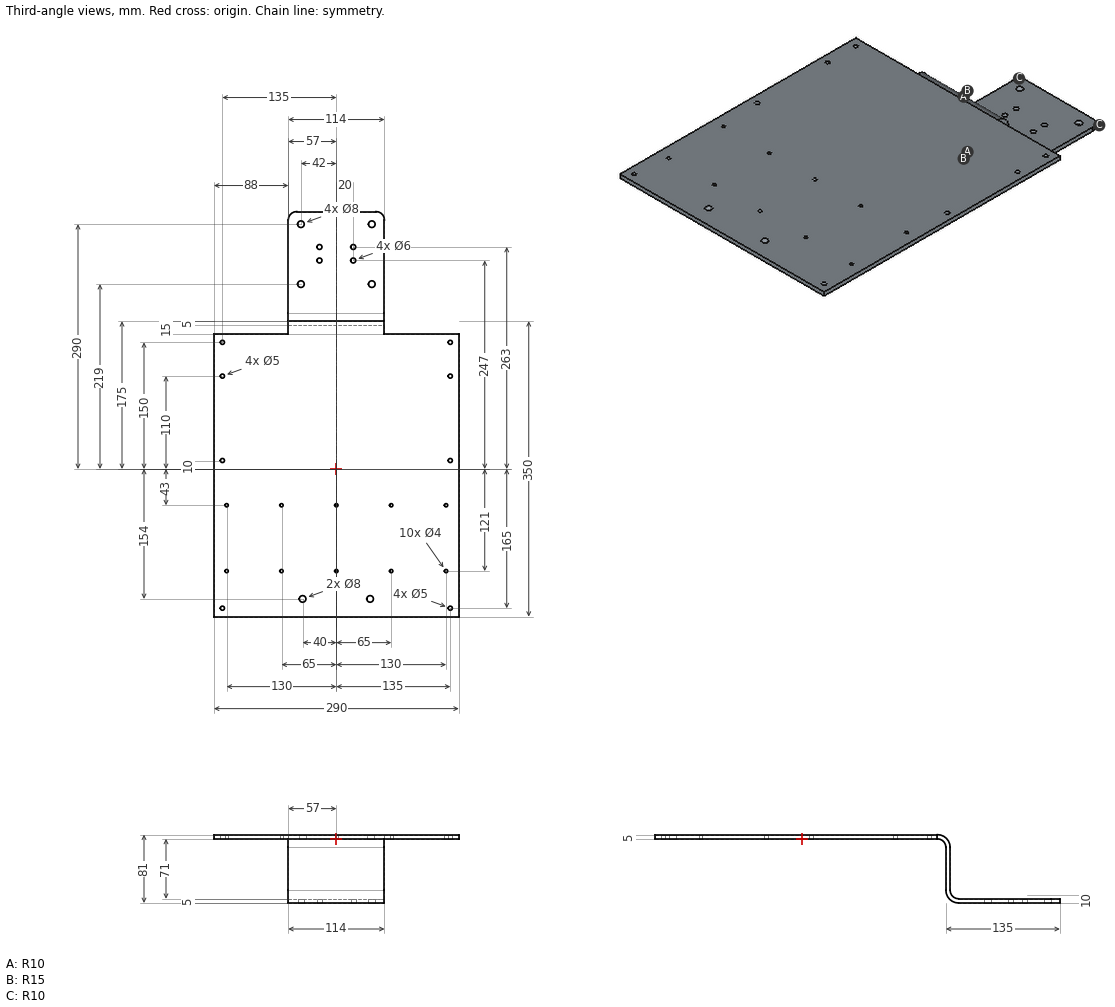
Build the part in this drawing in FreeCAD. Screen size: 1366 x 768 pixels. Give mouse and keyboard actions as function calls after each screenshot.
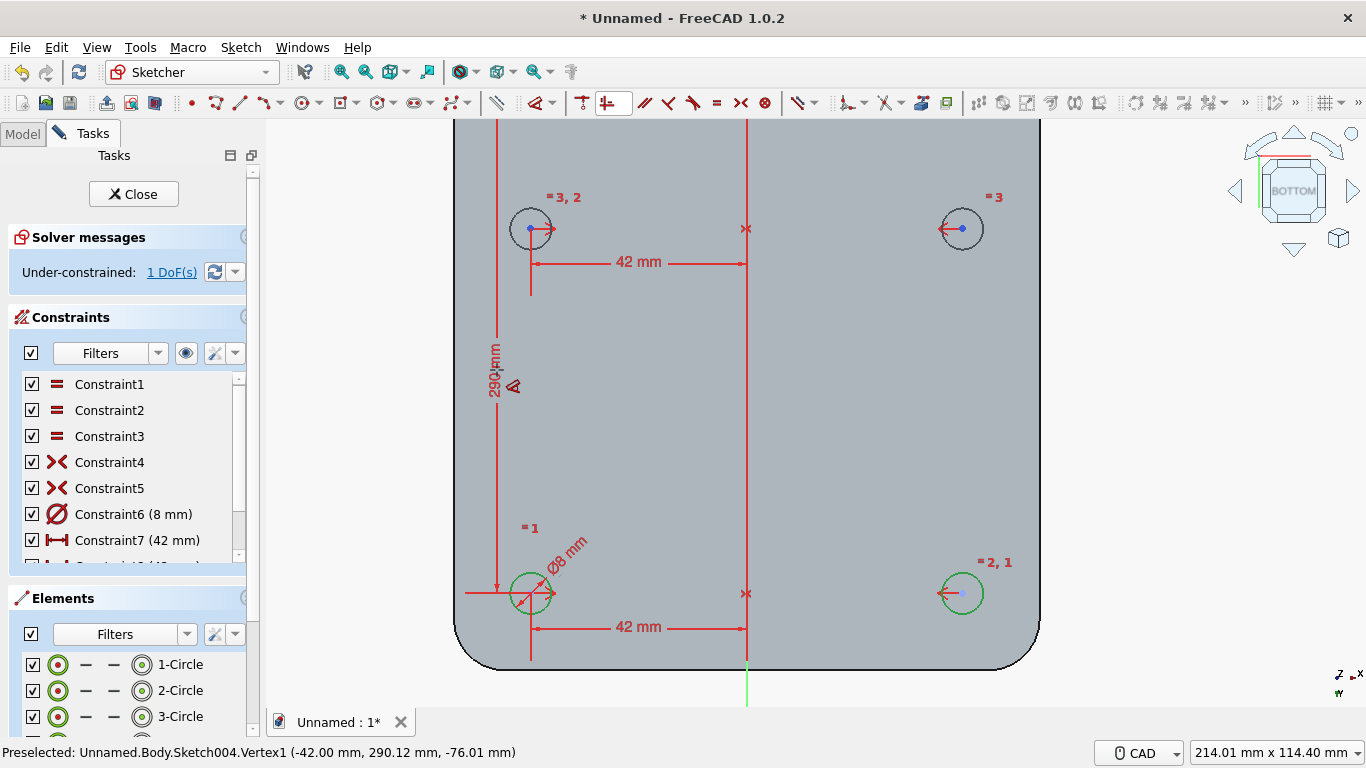
click(531, 229)
click(497, 188)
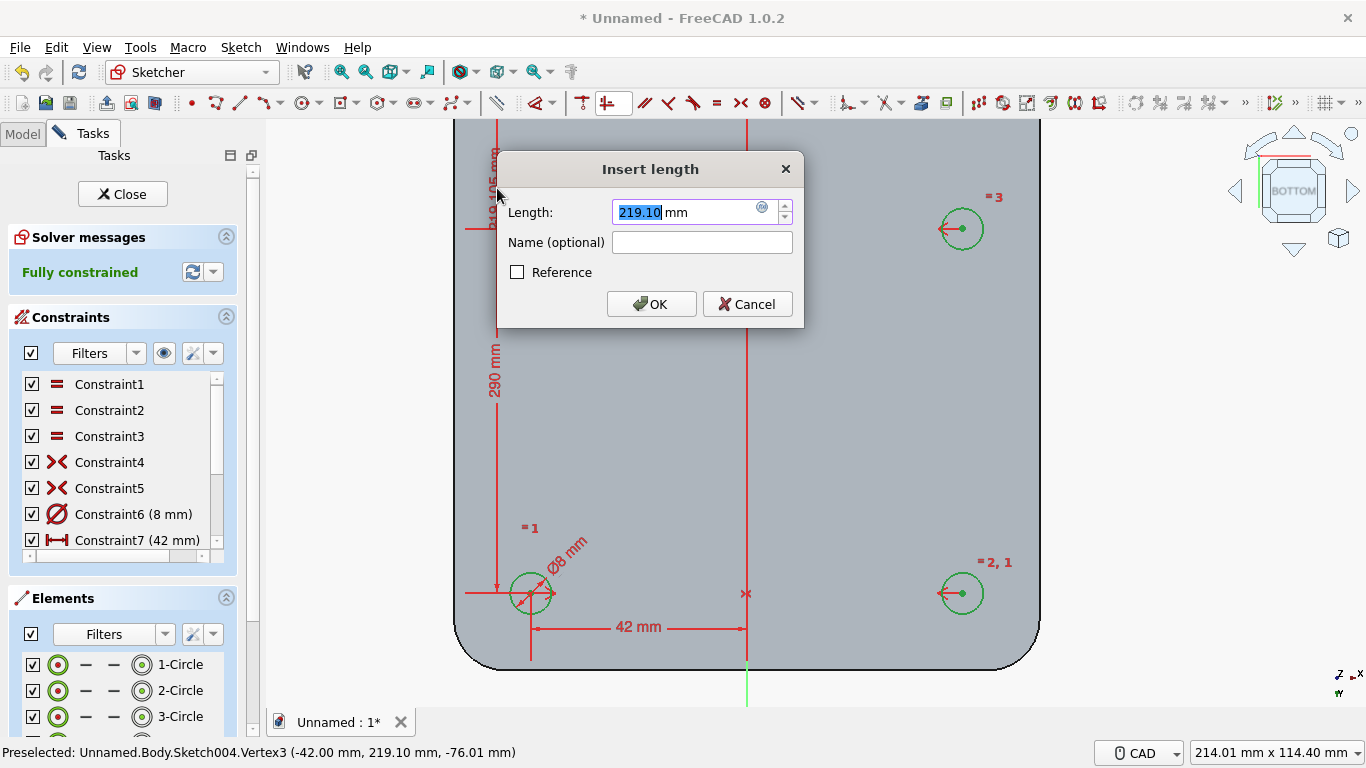
text(219)
key(Return)
key(Escape)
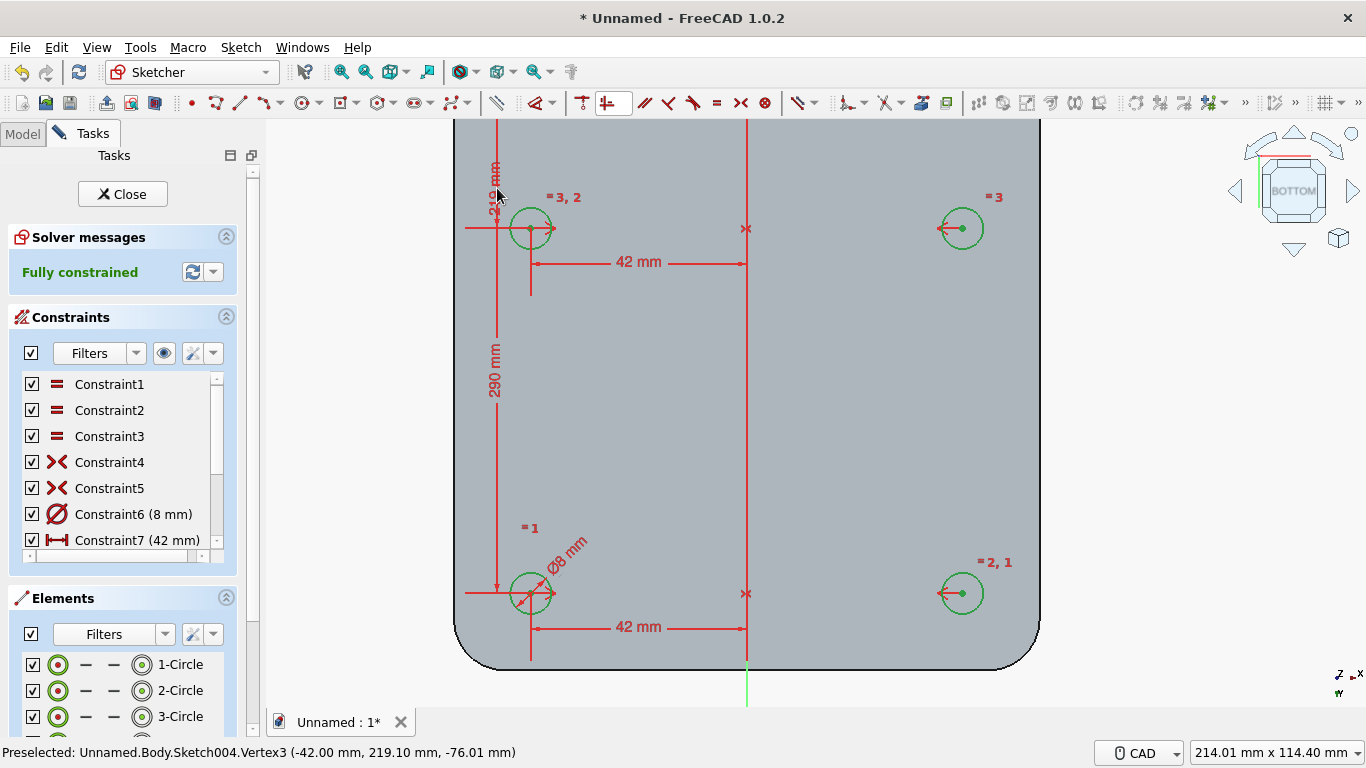
click(123, 194)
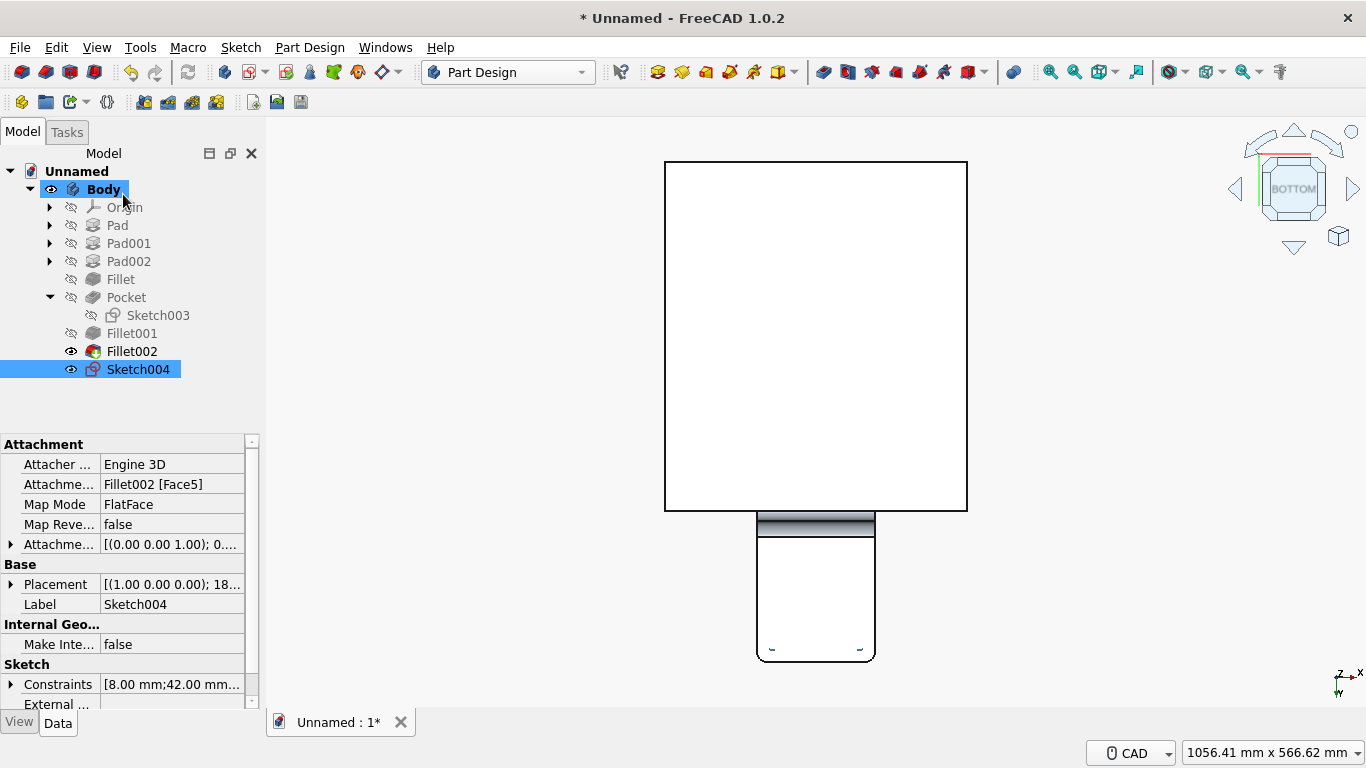
click(824, 72)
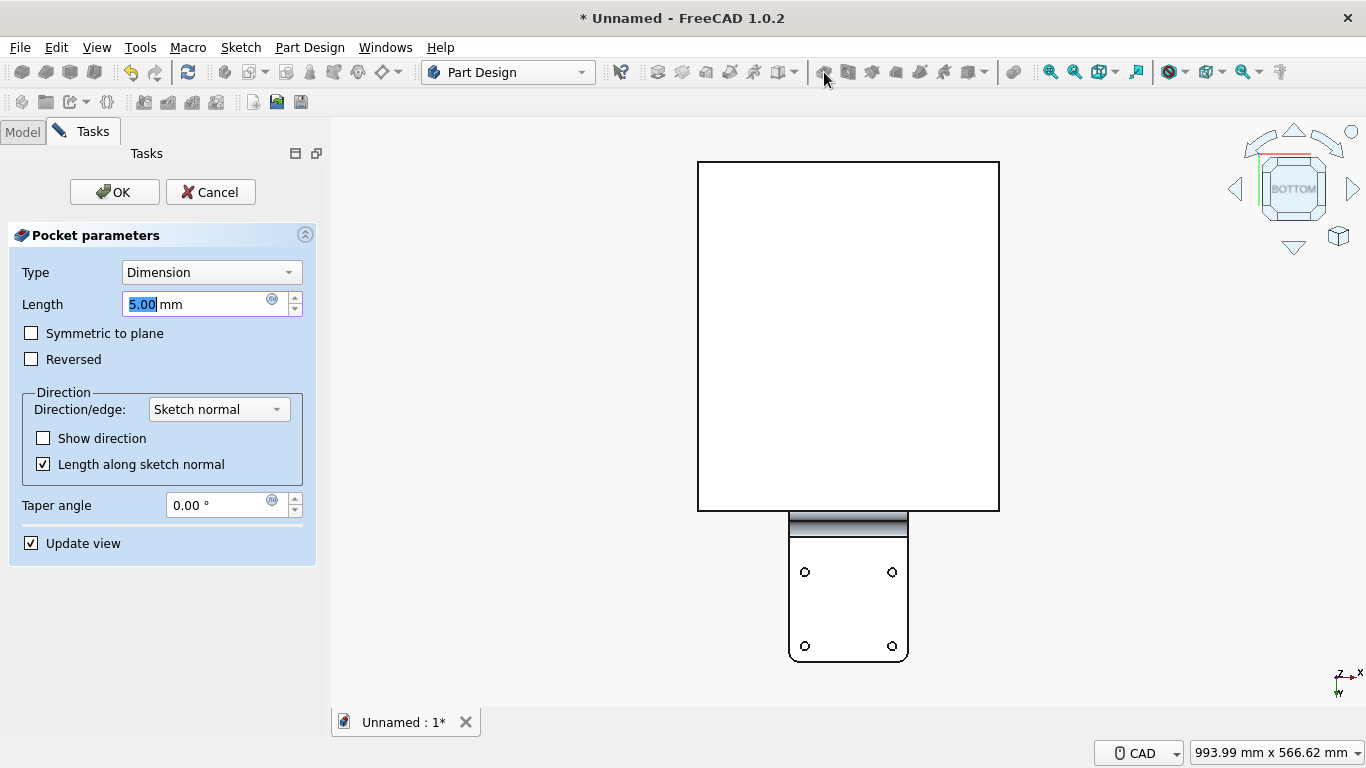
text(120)
key(Tab)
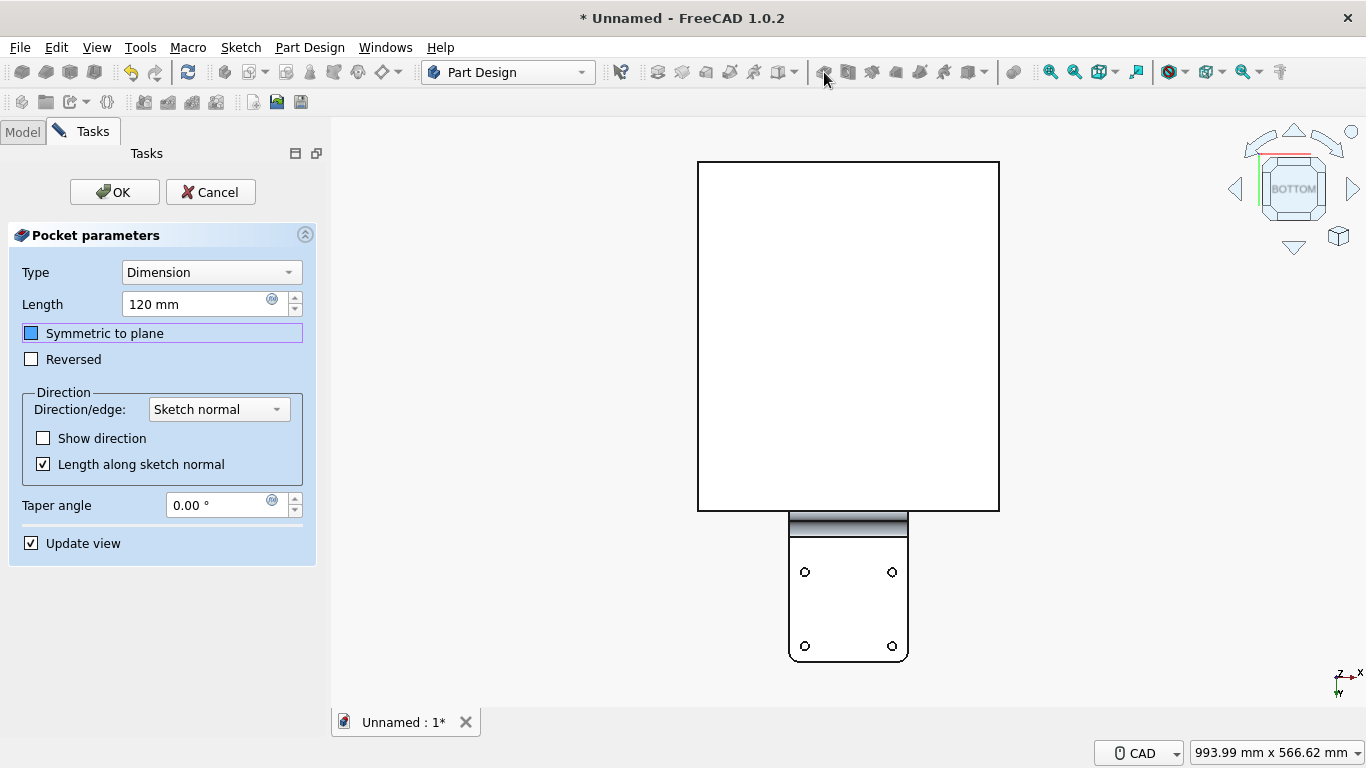
click(115, 192)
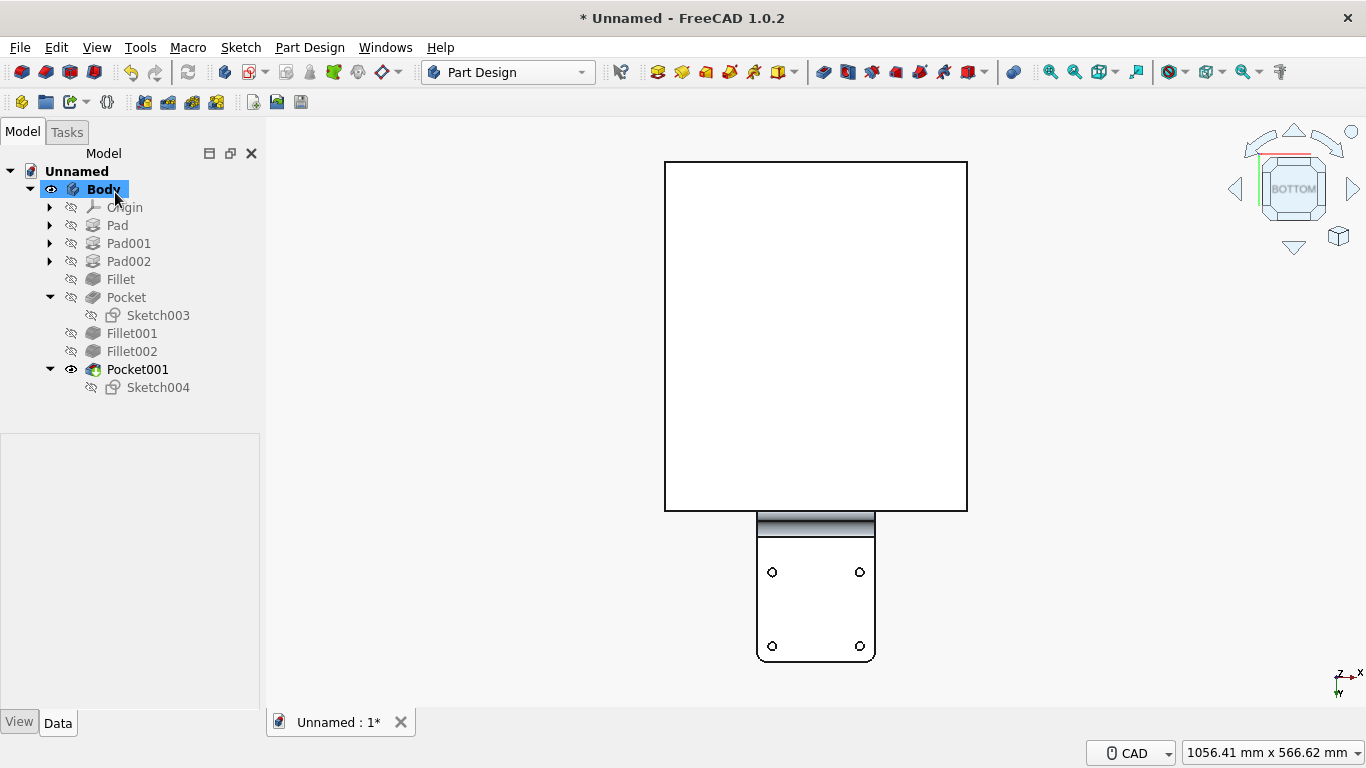
click(816, 336)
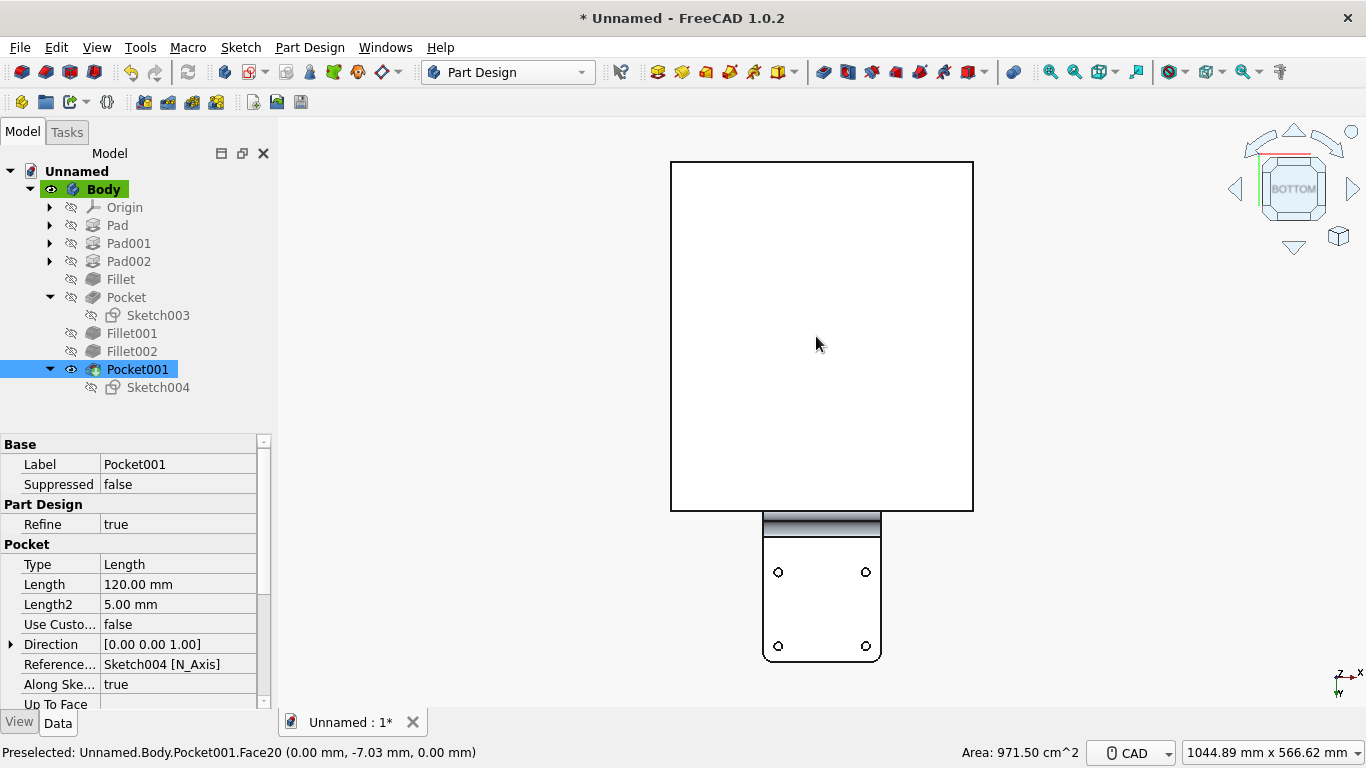
click(250, 72)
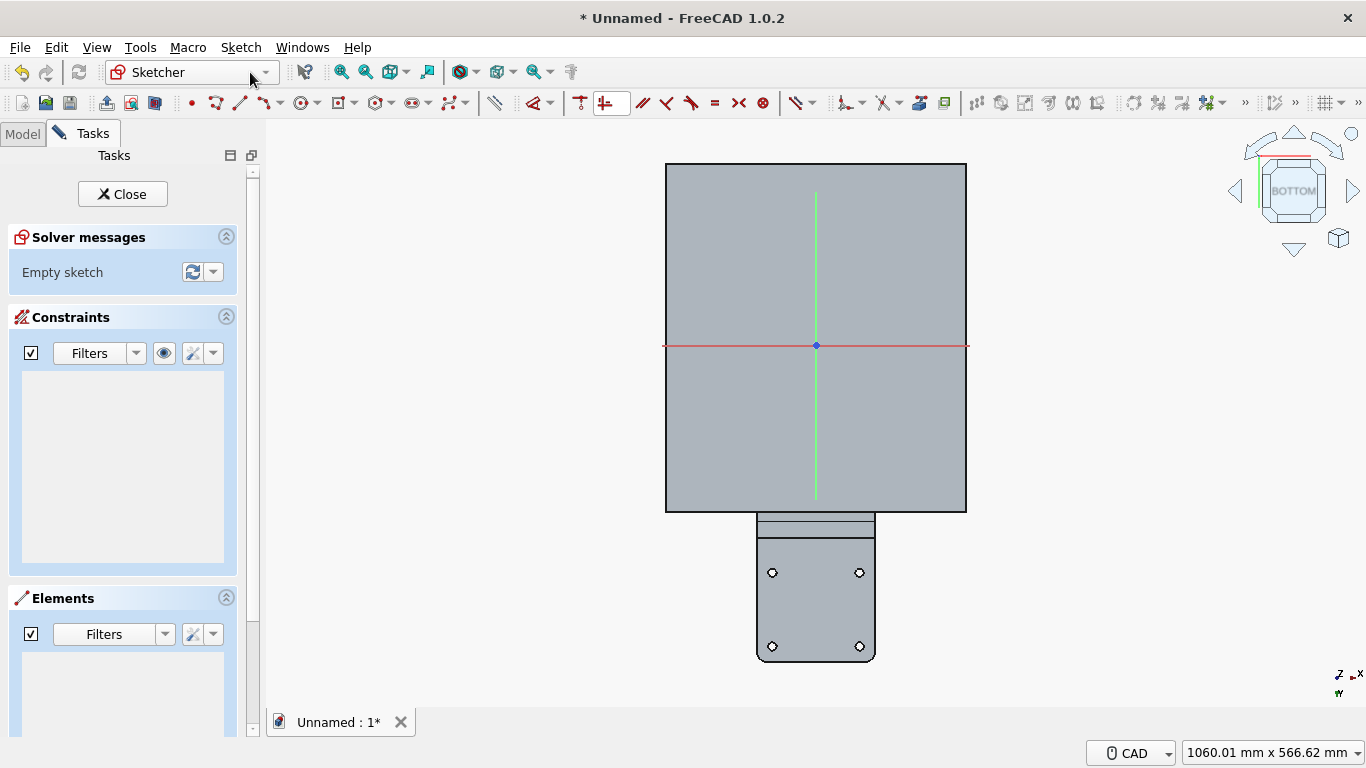
key(q)
key(s)